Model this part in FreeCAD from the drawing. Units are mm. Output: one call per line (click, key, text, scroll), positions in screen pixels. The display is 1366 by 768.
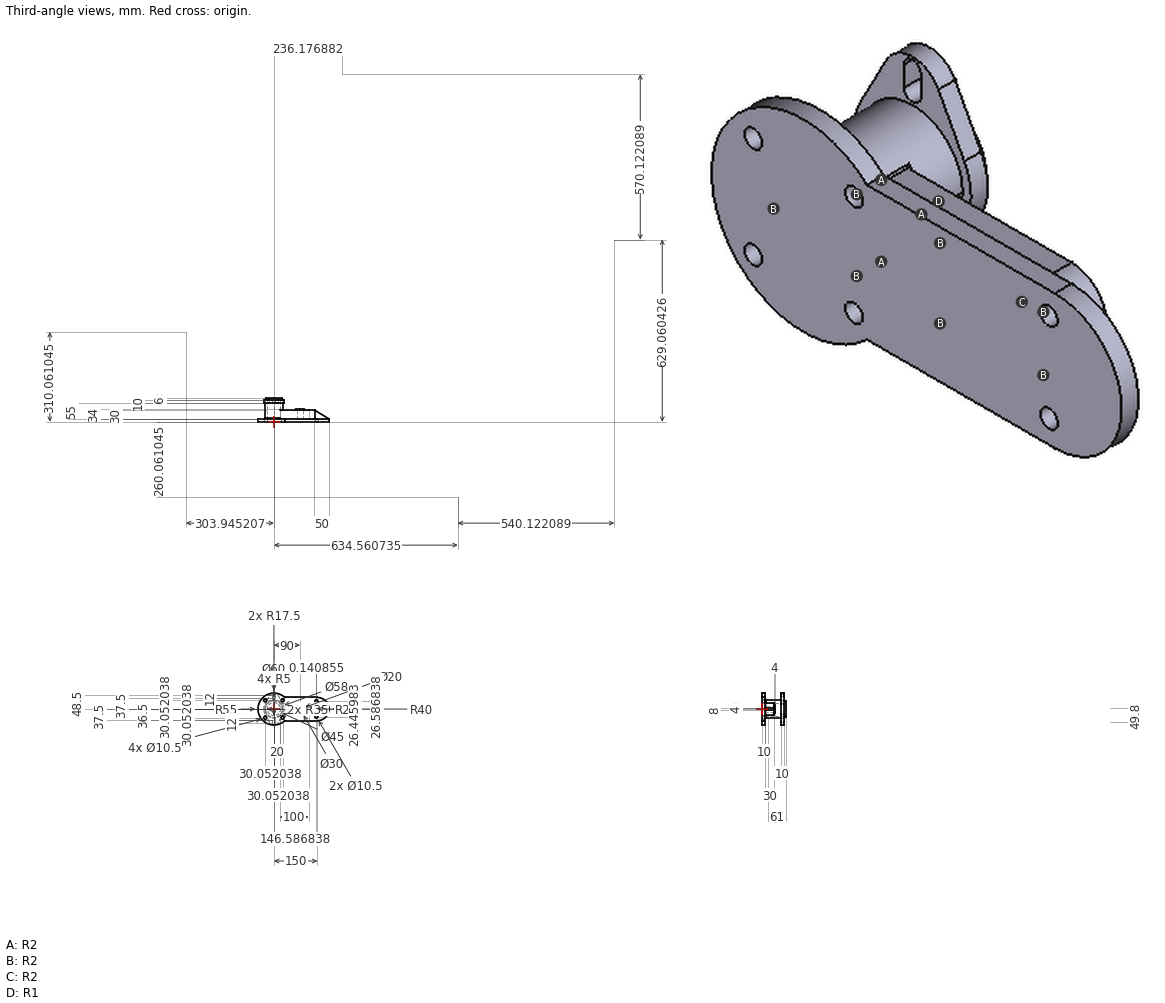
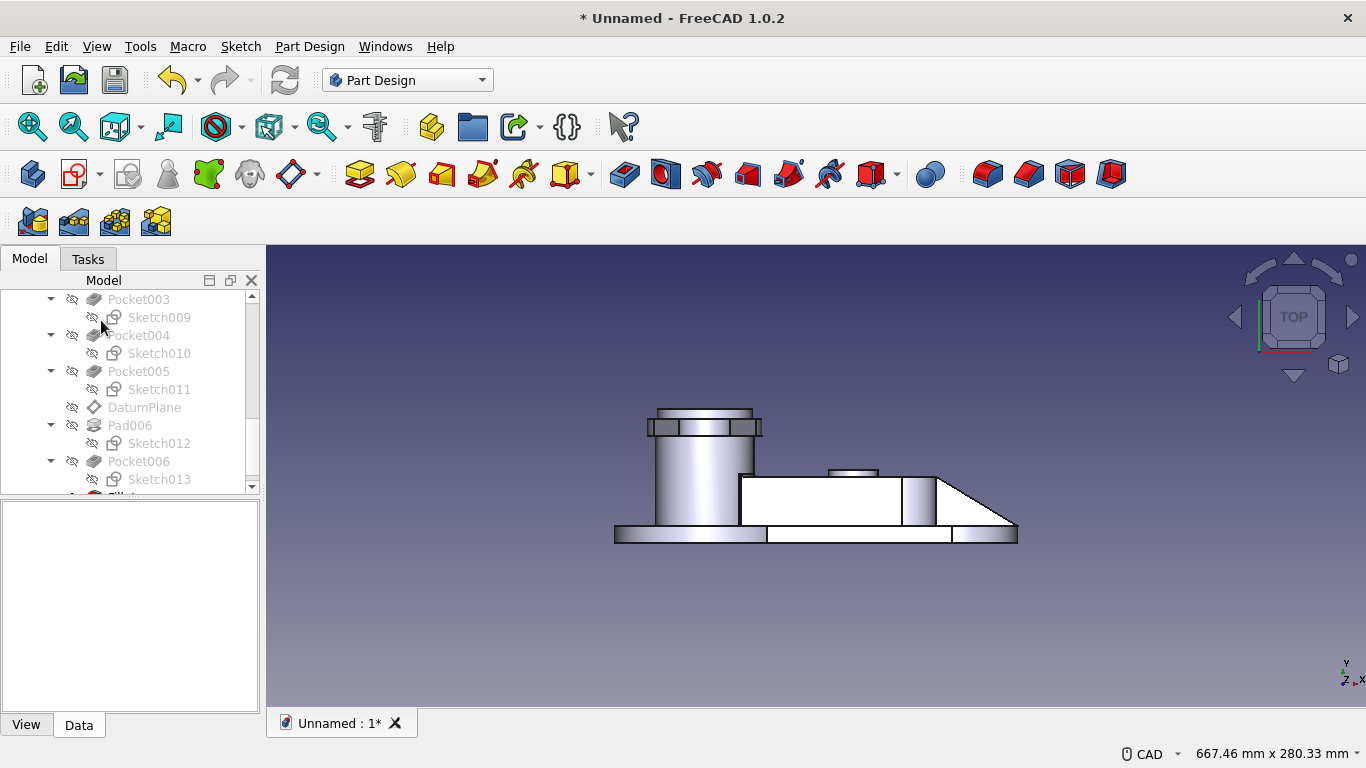
key(v)
key(f)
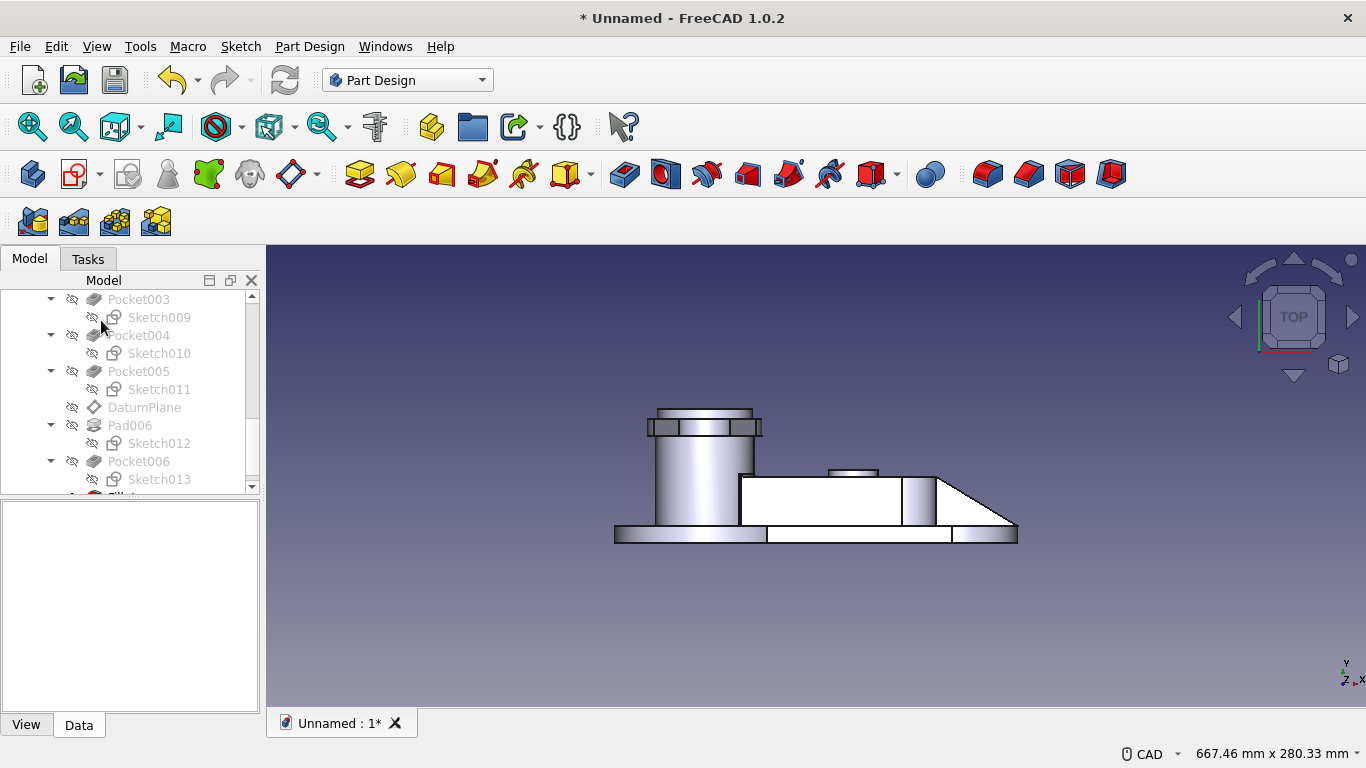
key(0)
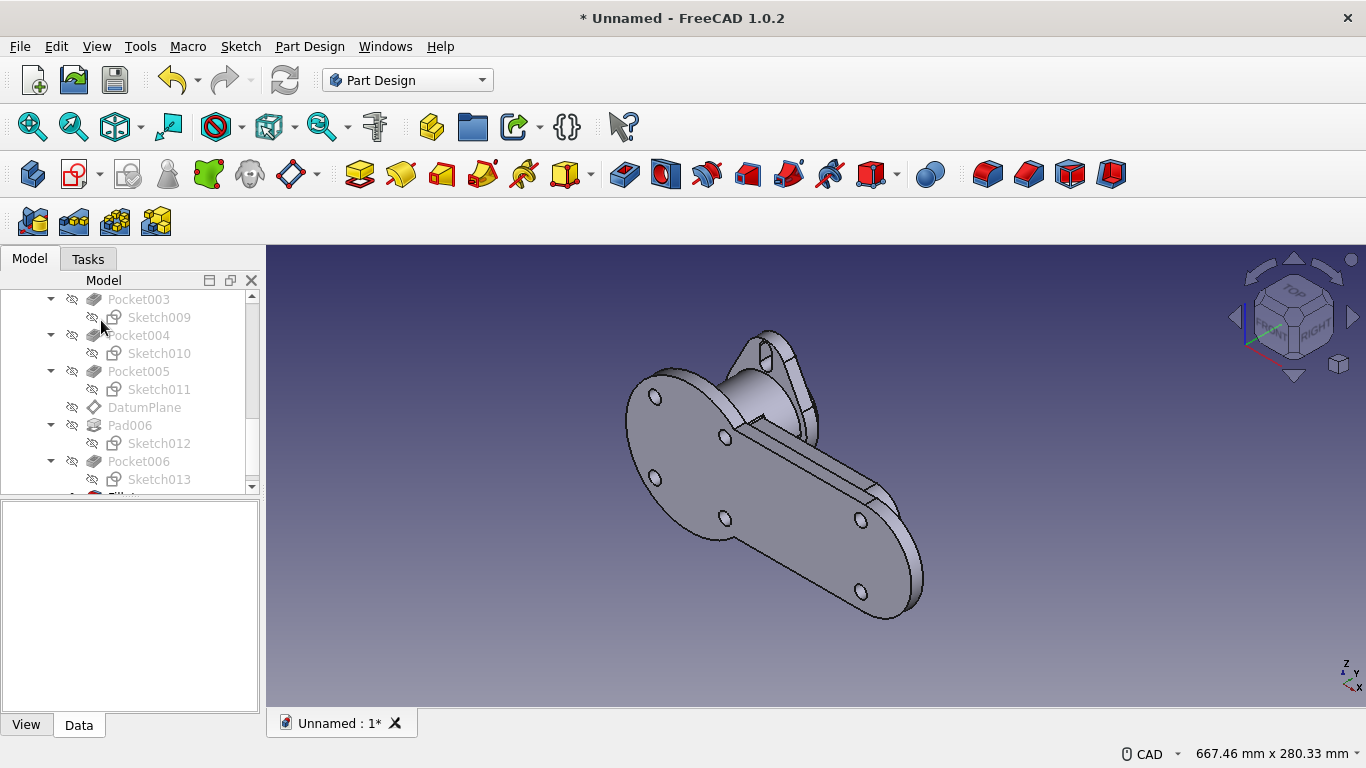
key(1)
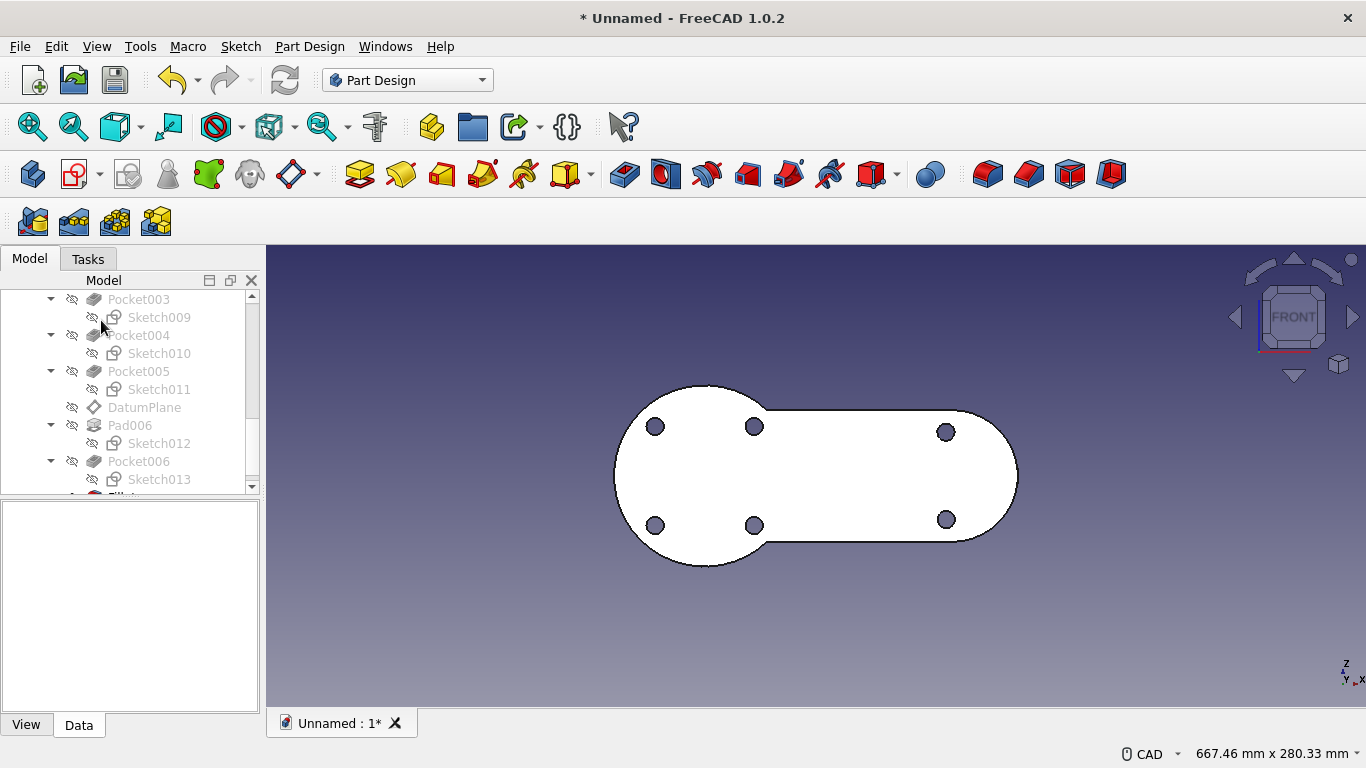
key(v)
key(f)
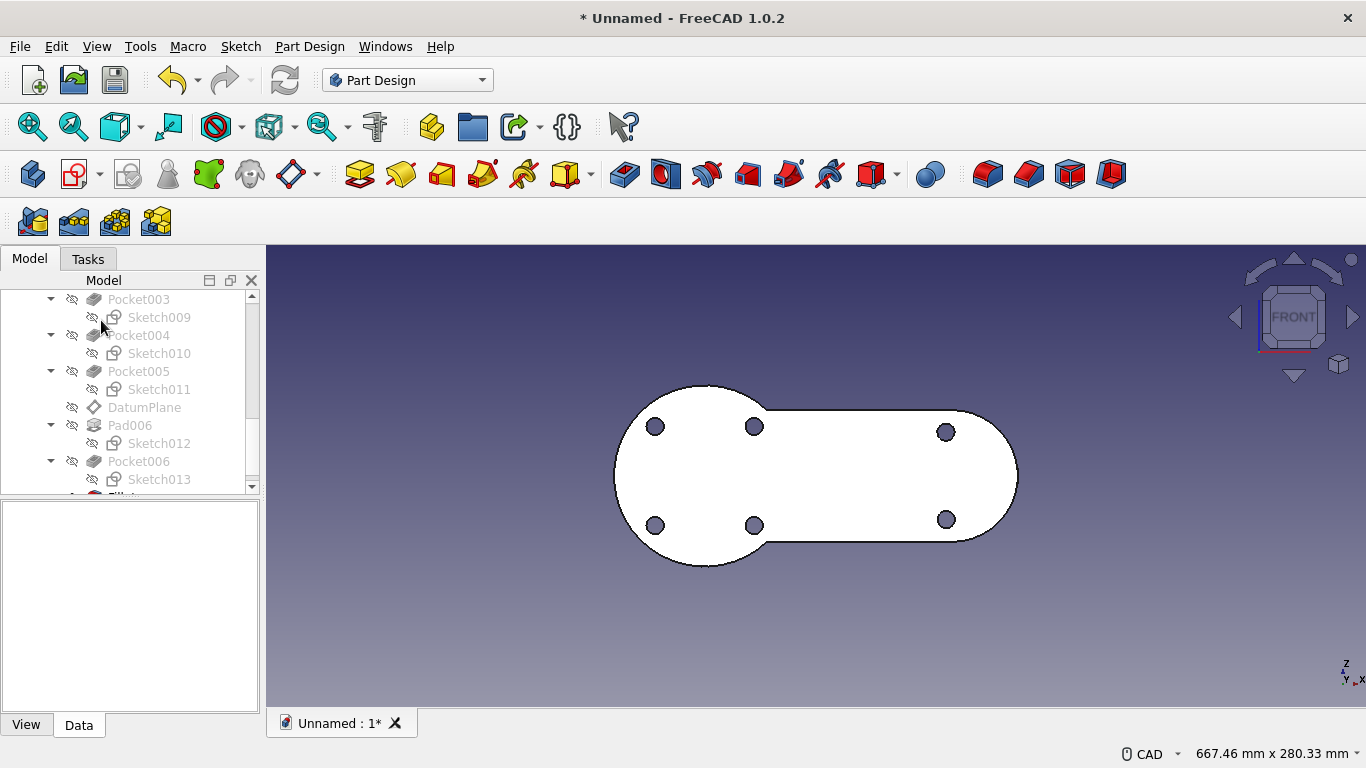
key(3)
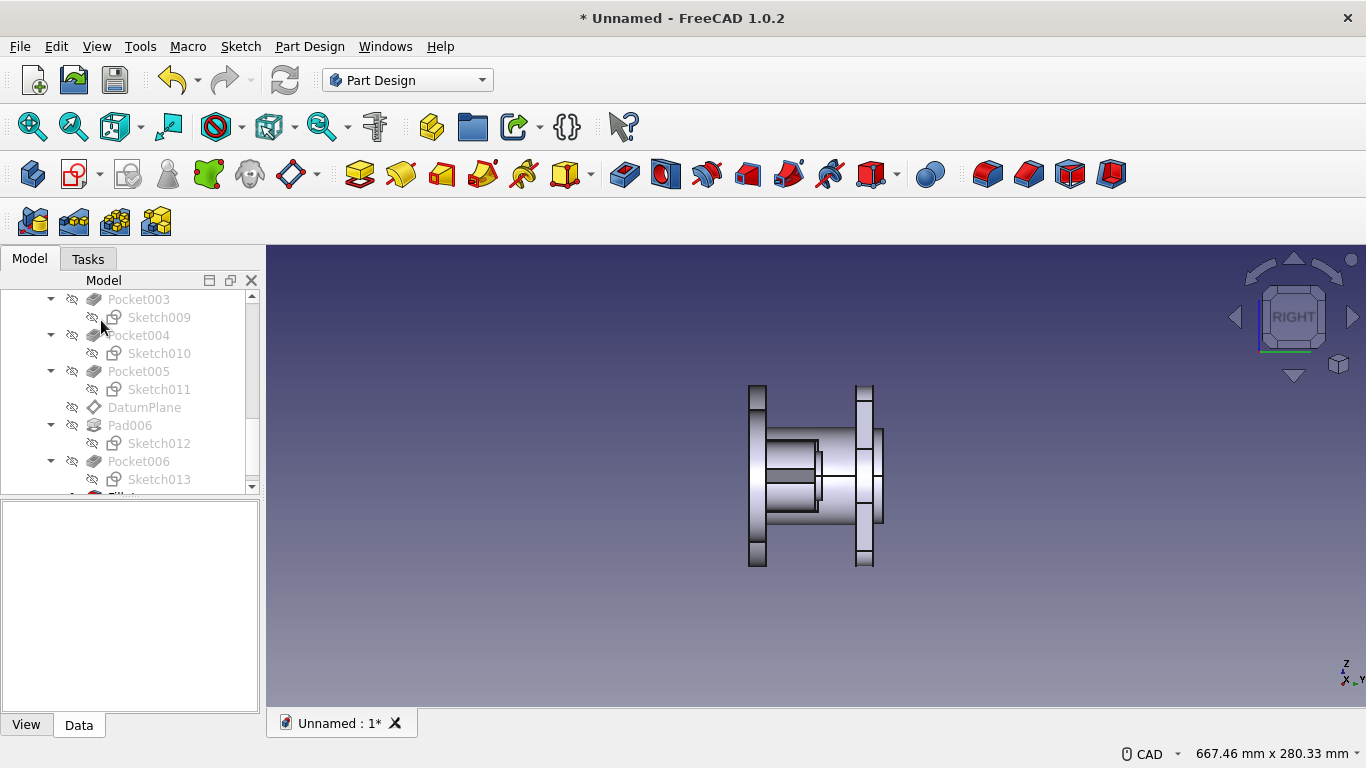
click(33, 128)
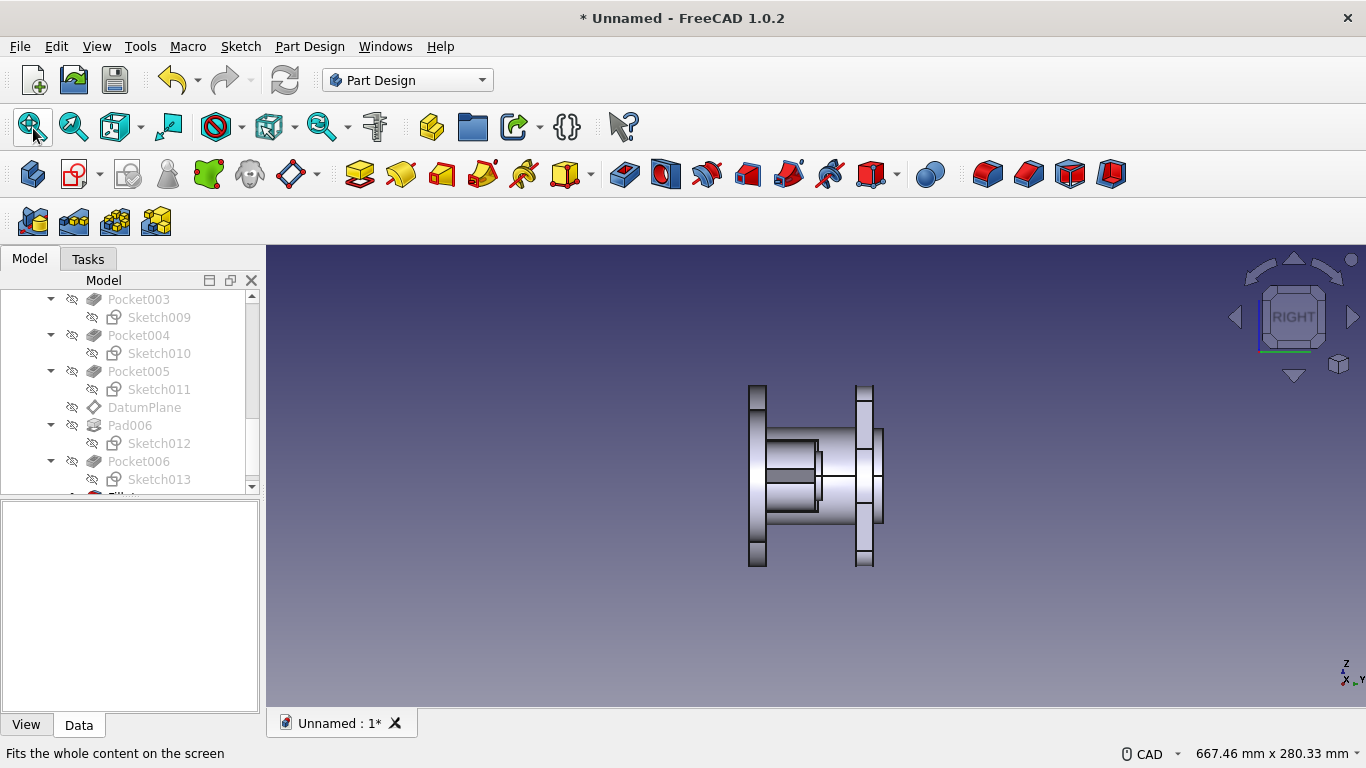
key(5)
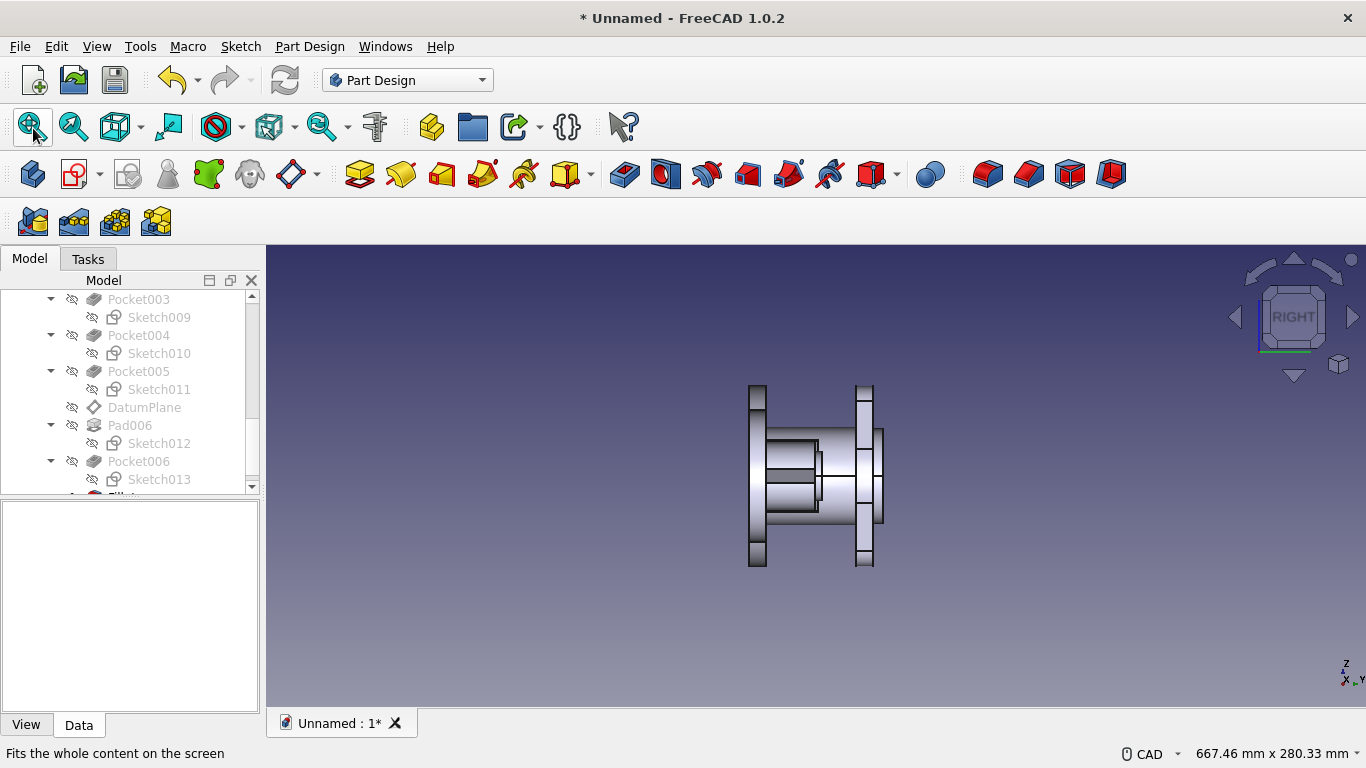
key(v)
key(f)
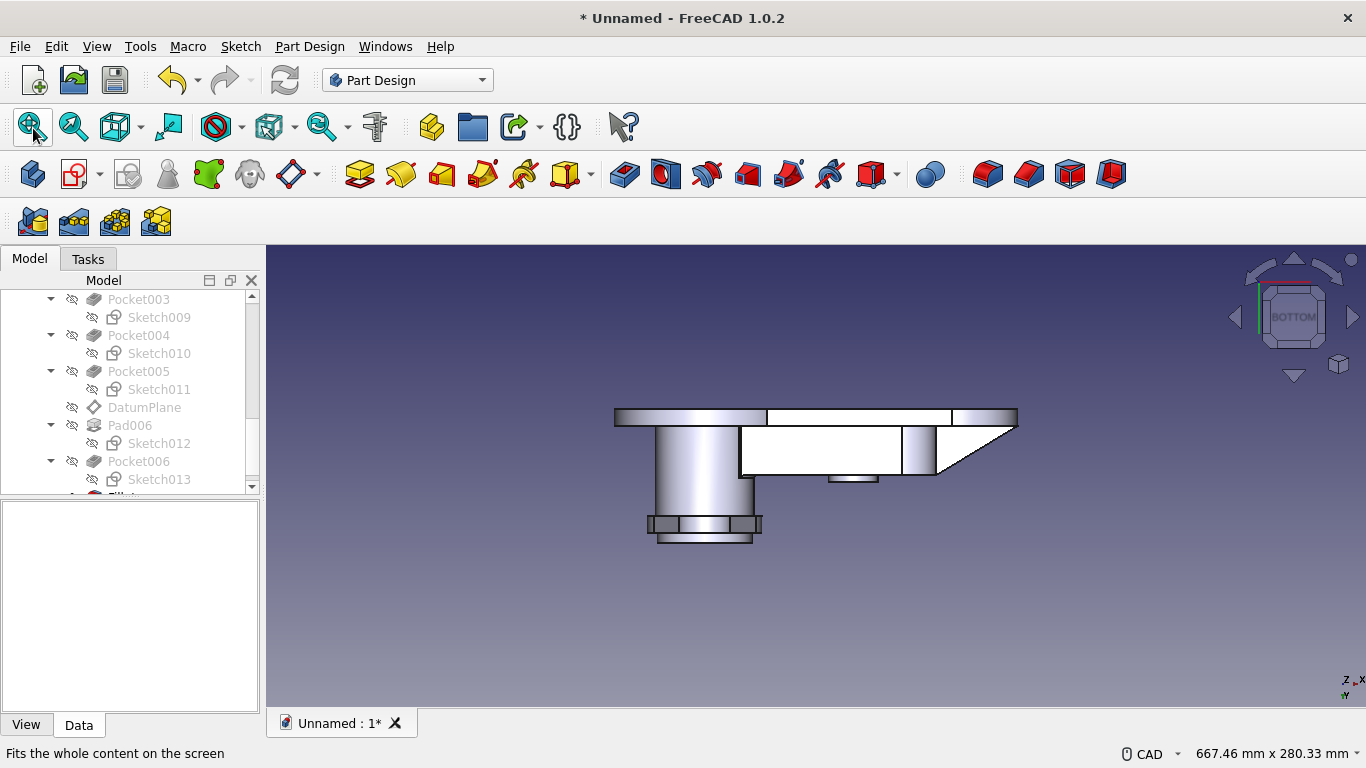
key(4)